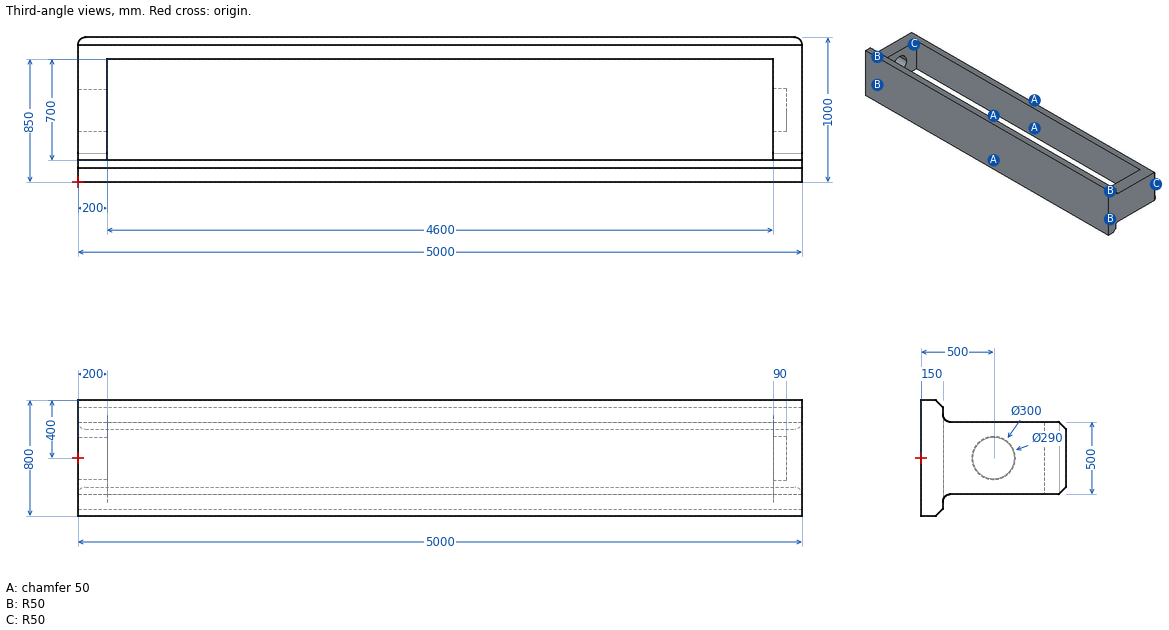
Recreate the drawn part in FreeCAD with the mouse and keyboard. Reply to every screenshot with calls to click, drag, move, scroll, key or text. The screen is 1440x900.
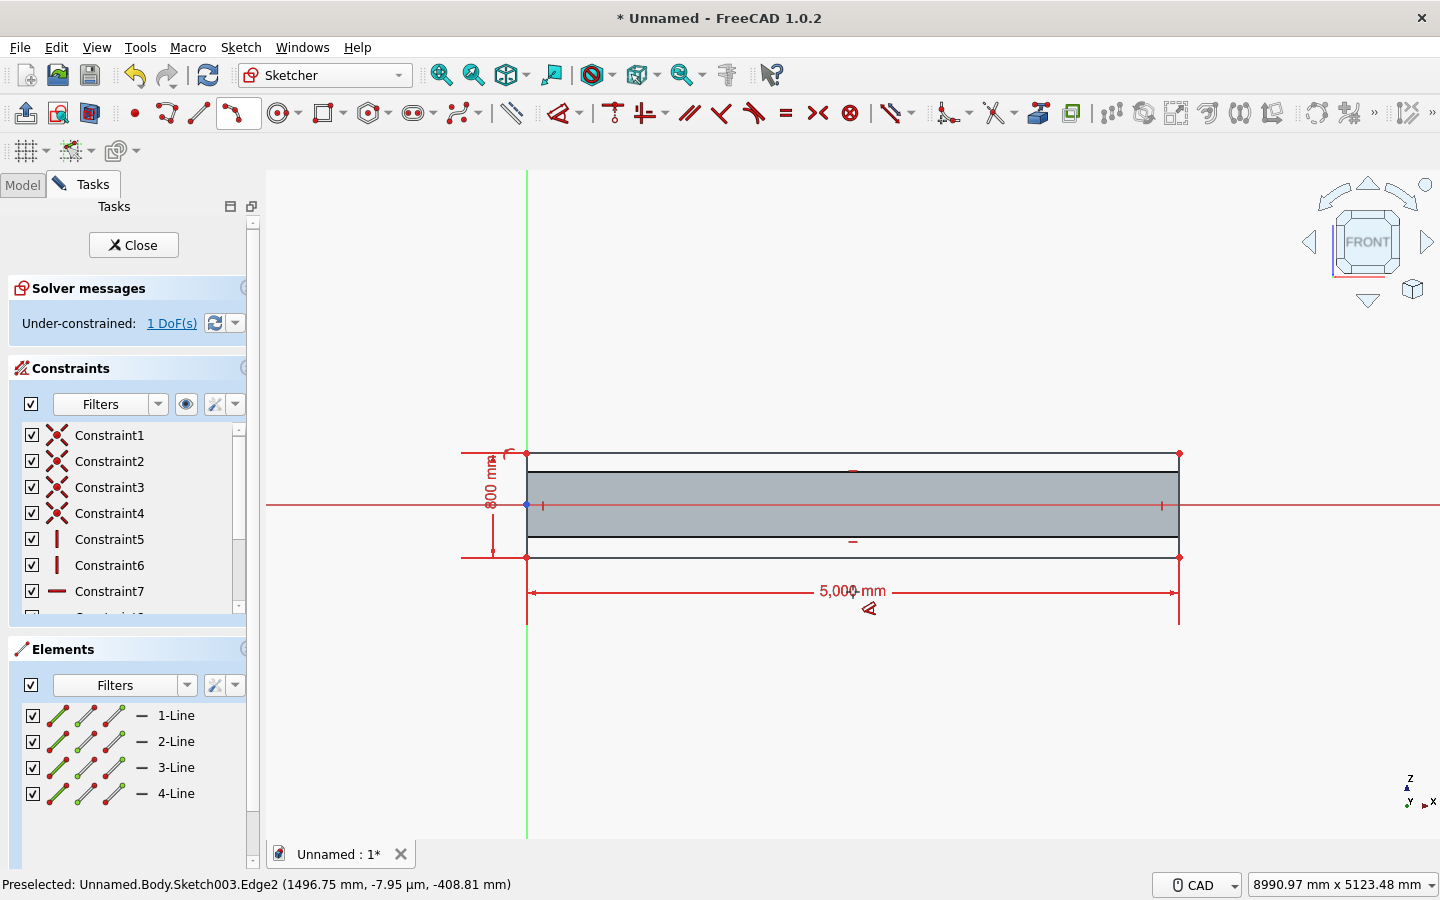
click(527, 453)
click(493, 461)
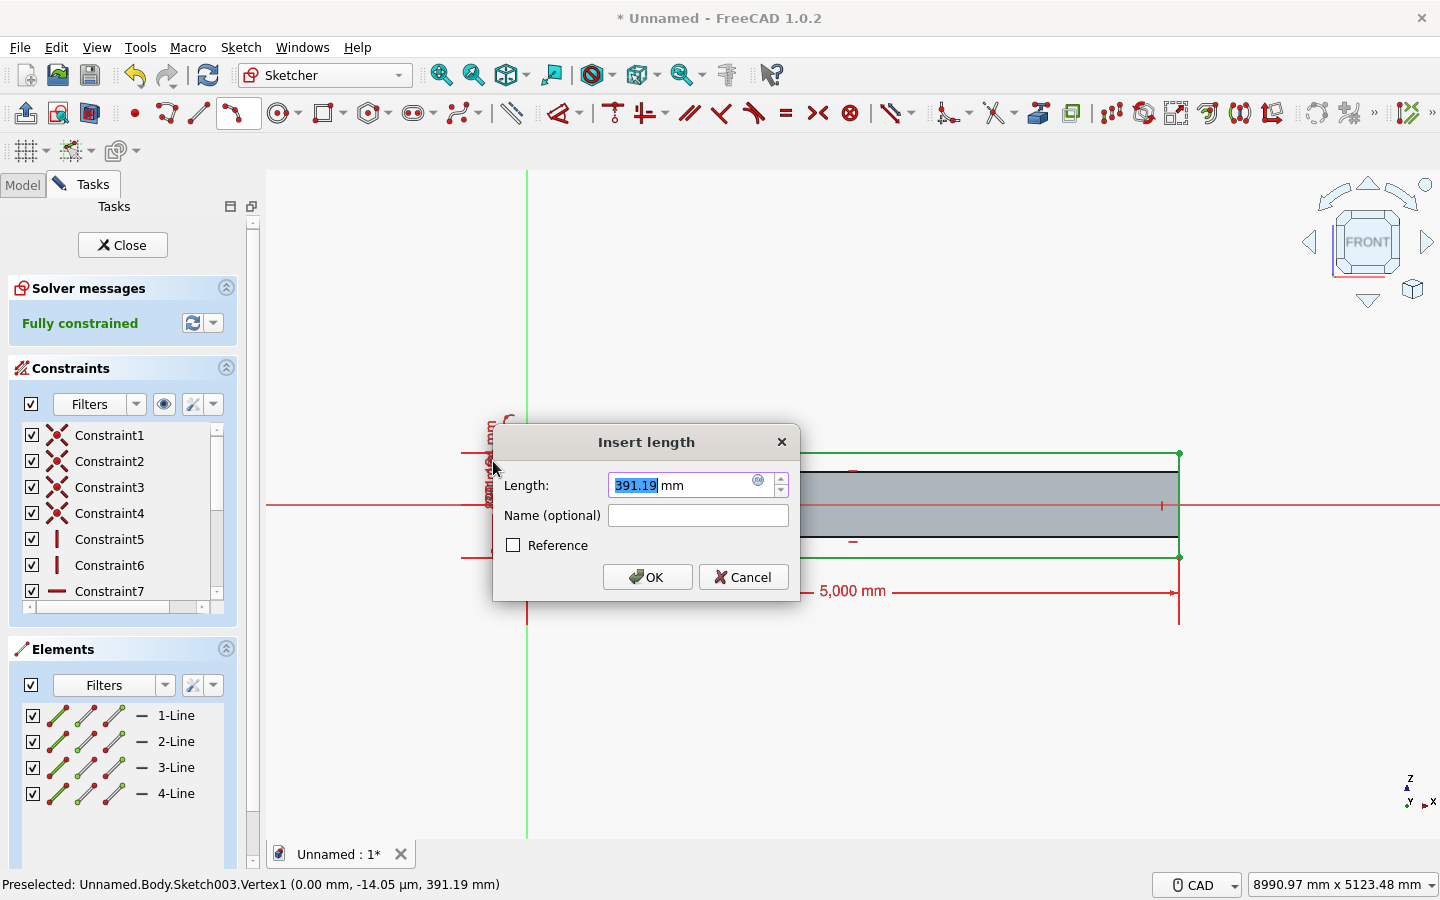
text(400)
key(Return)
key(Escape)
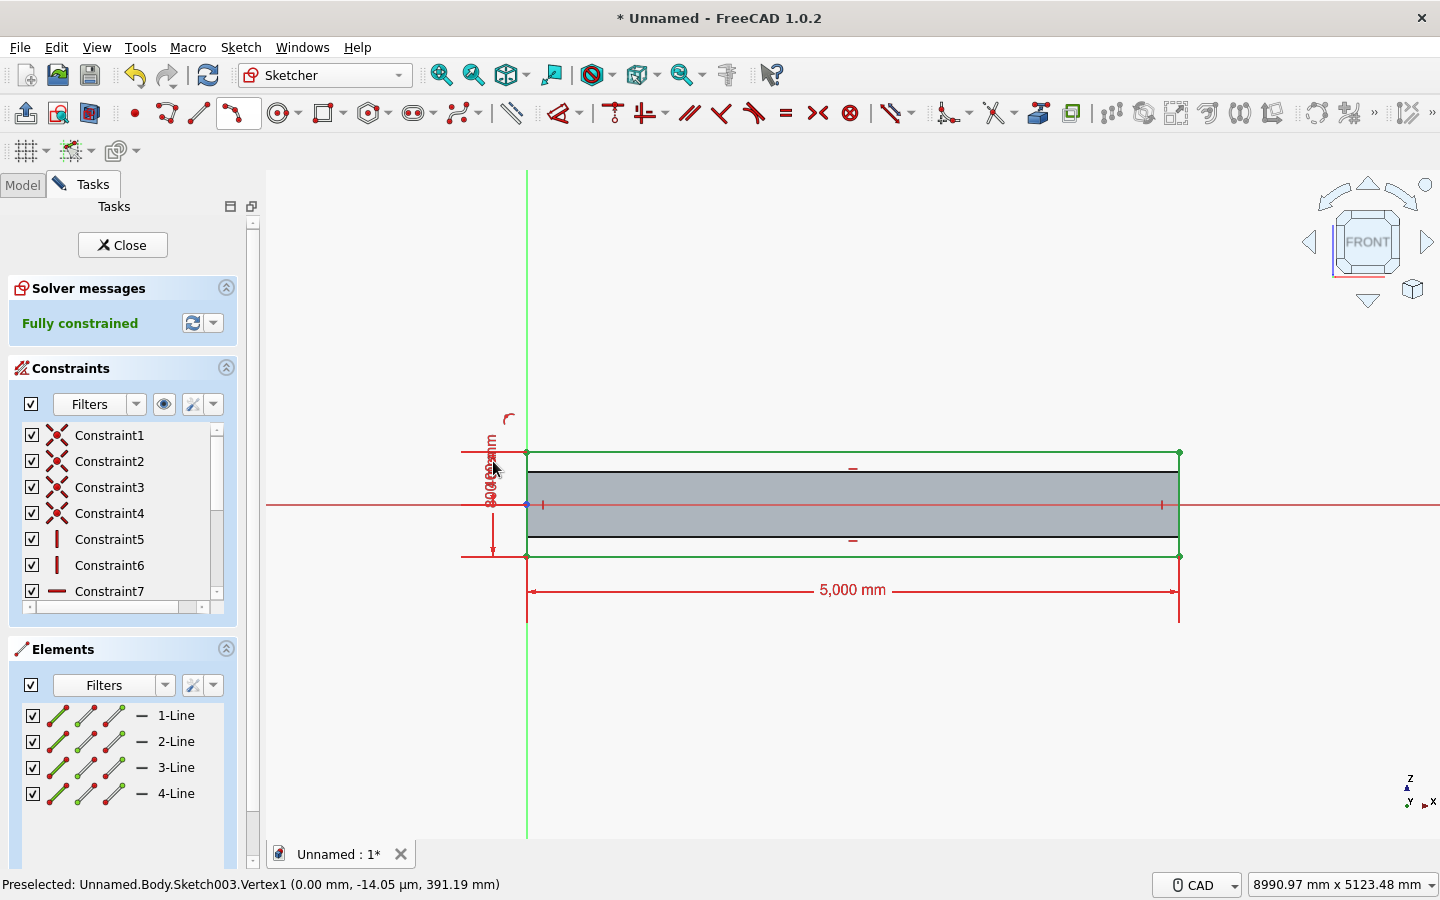
click(123, 245)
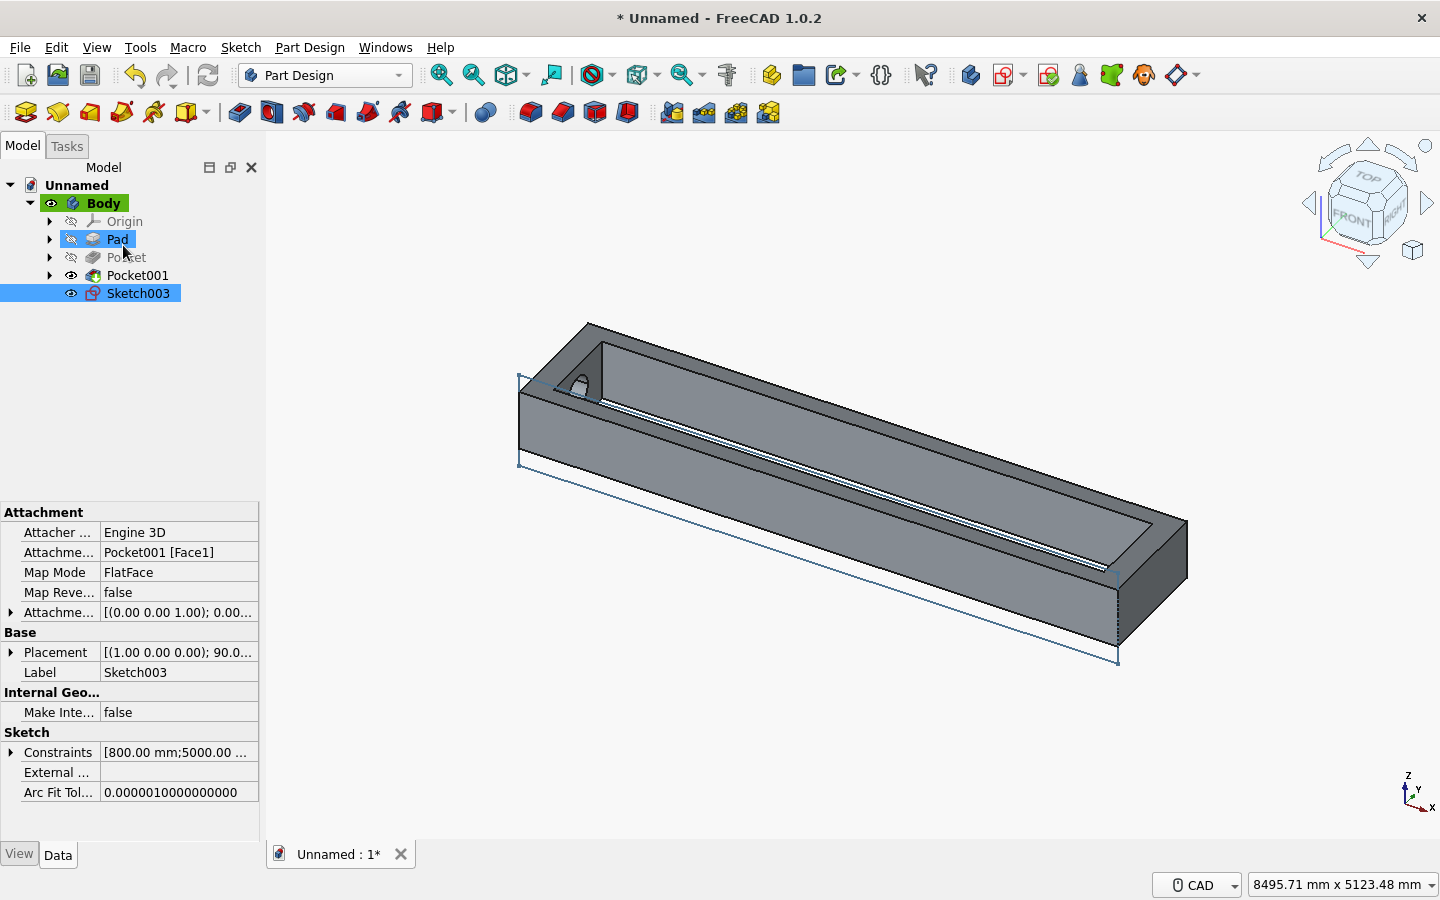
click(26, 112)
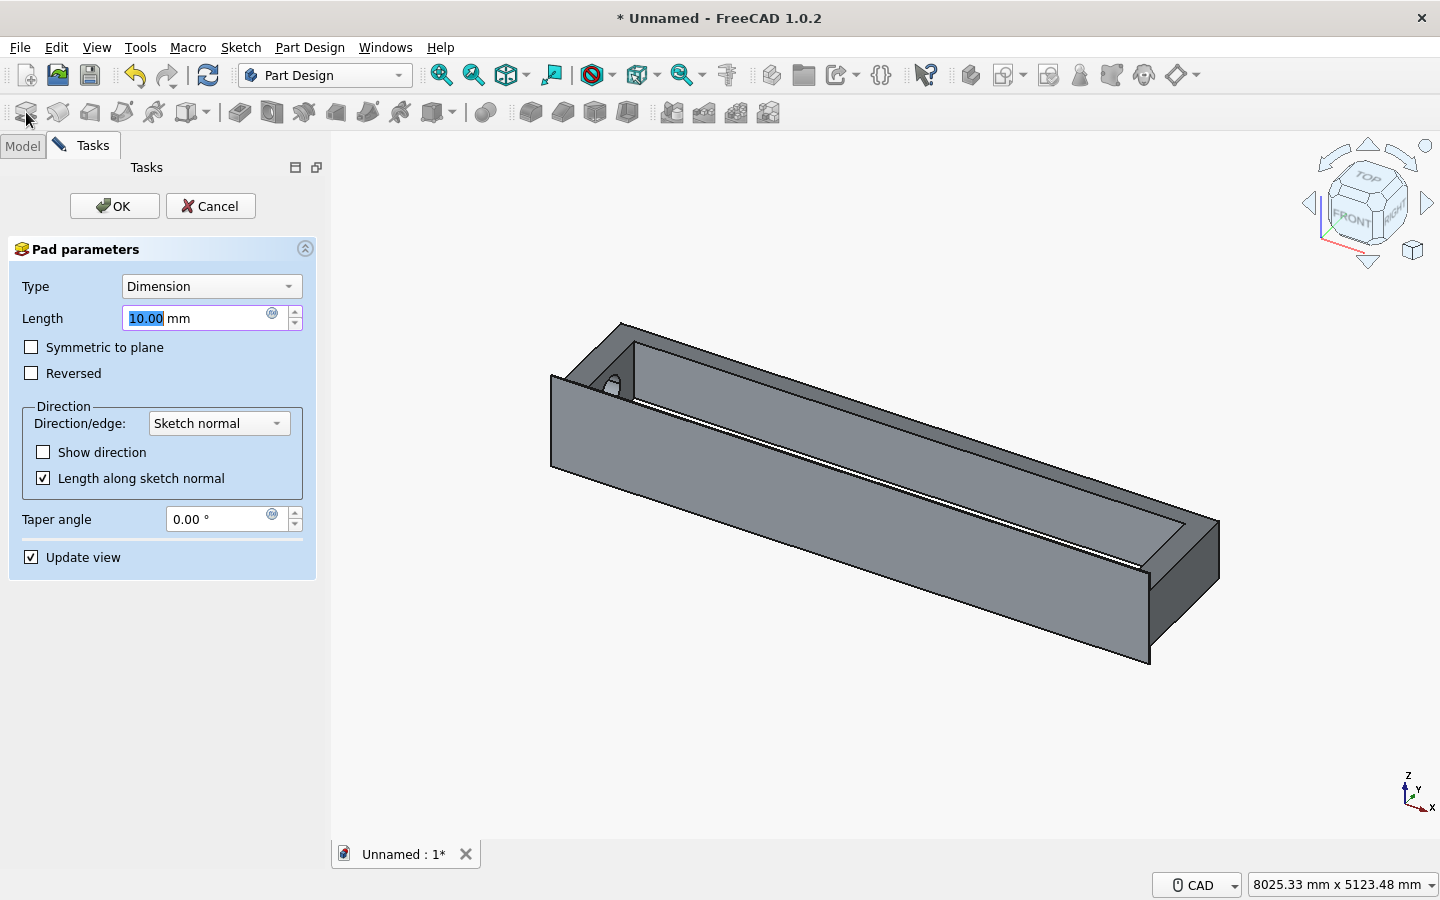
text(150)
key(Tab)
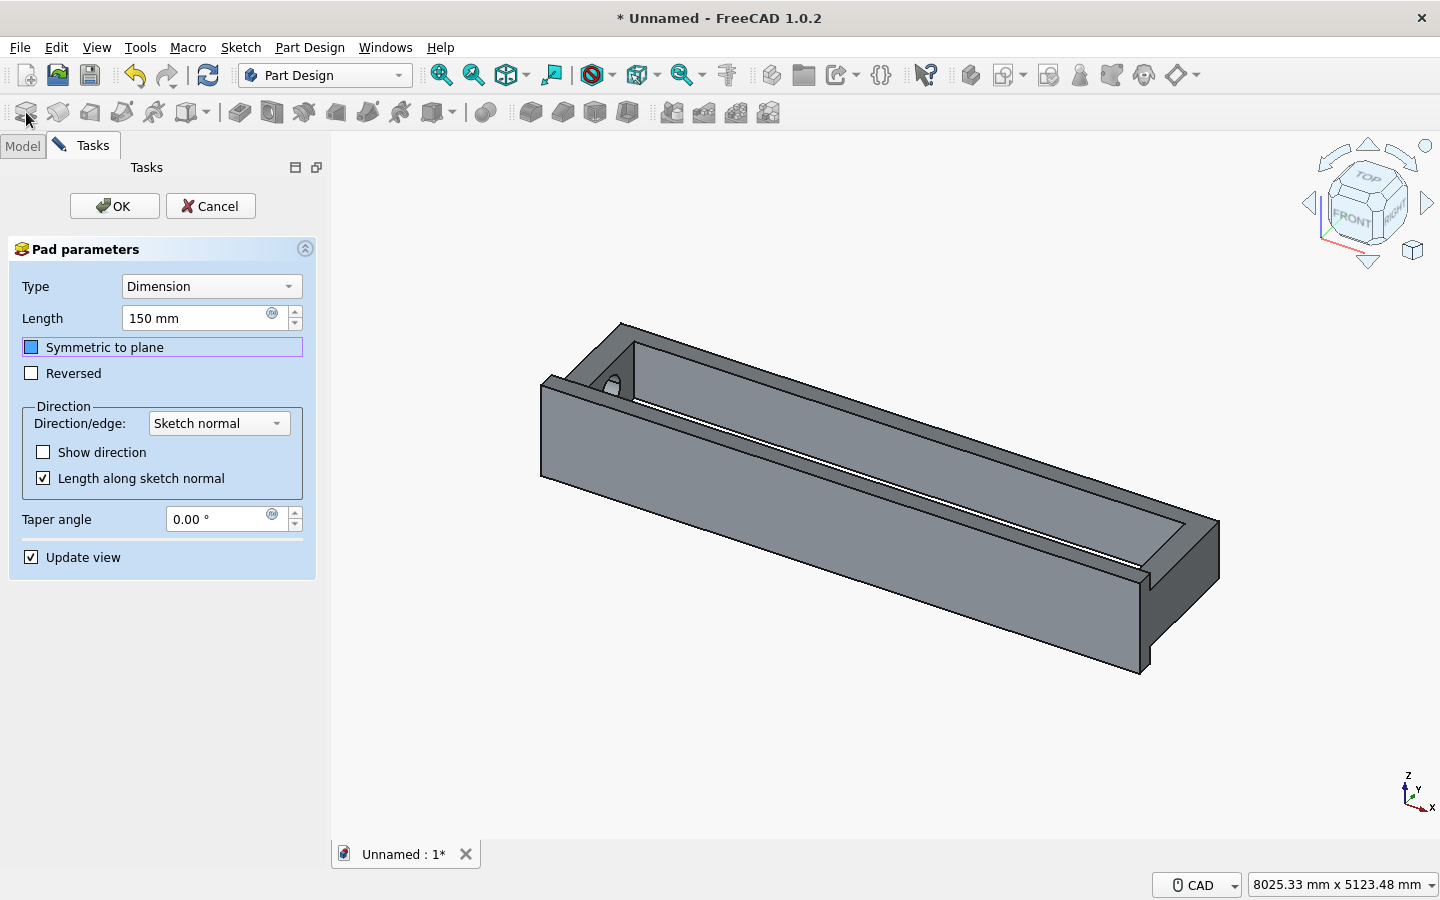
click(30, 373)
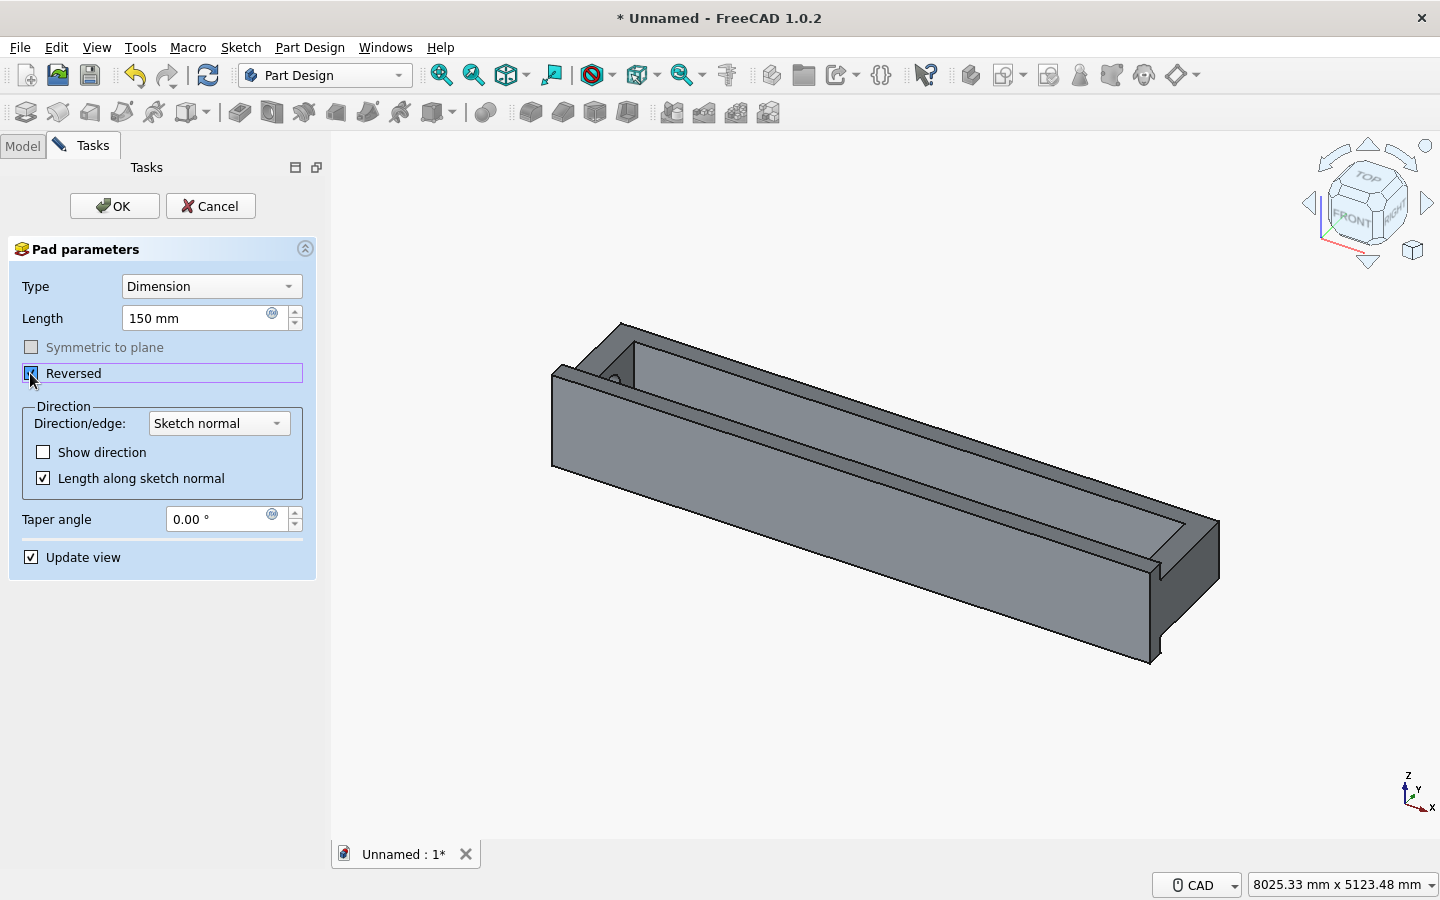
click(115, 206)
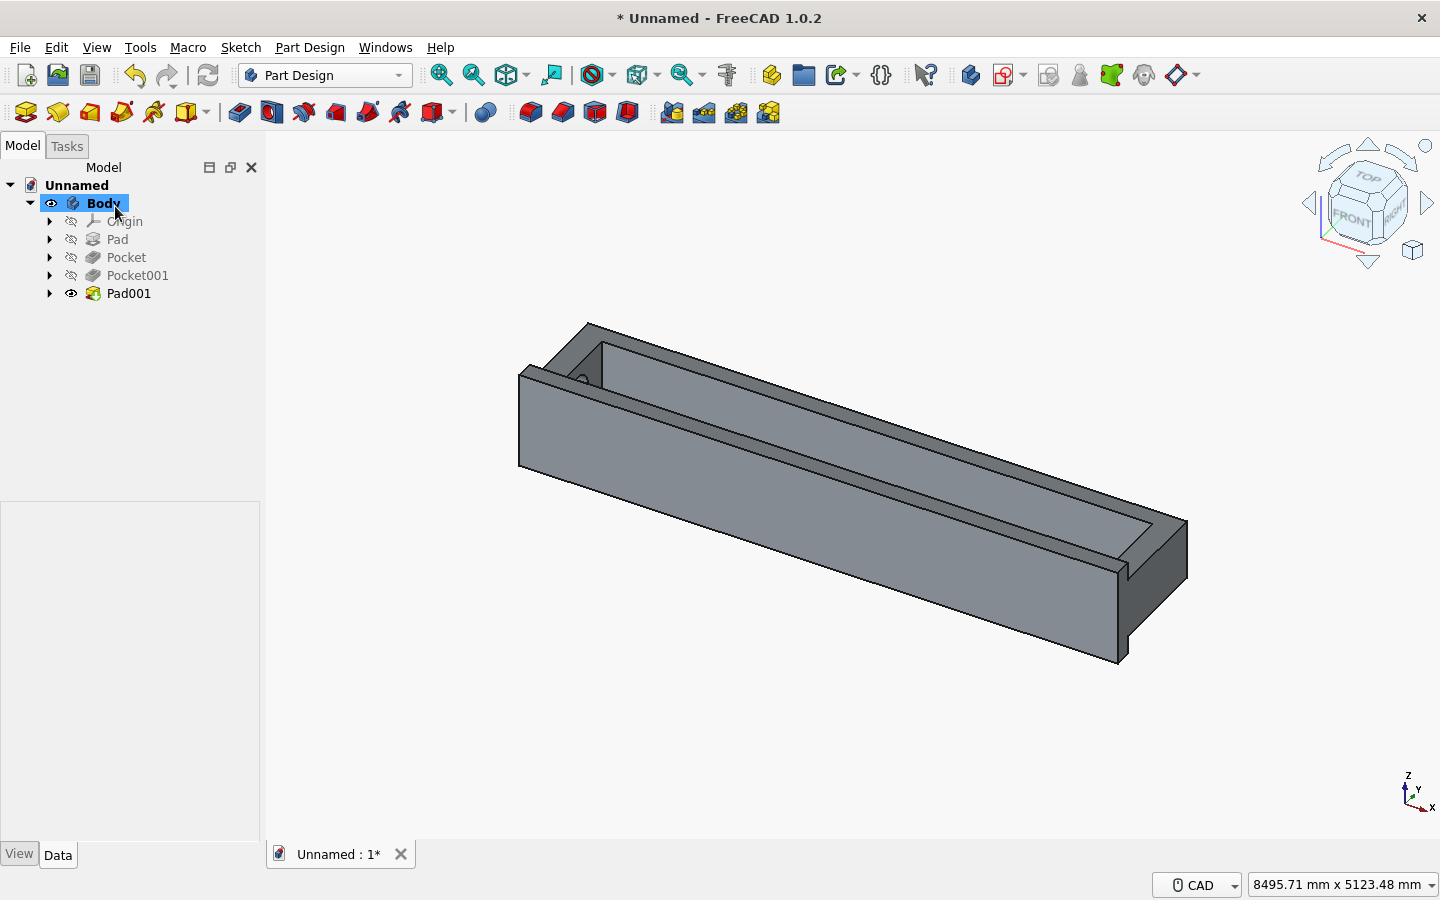
key(0)